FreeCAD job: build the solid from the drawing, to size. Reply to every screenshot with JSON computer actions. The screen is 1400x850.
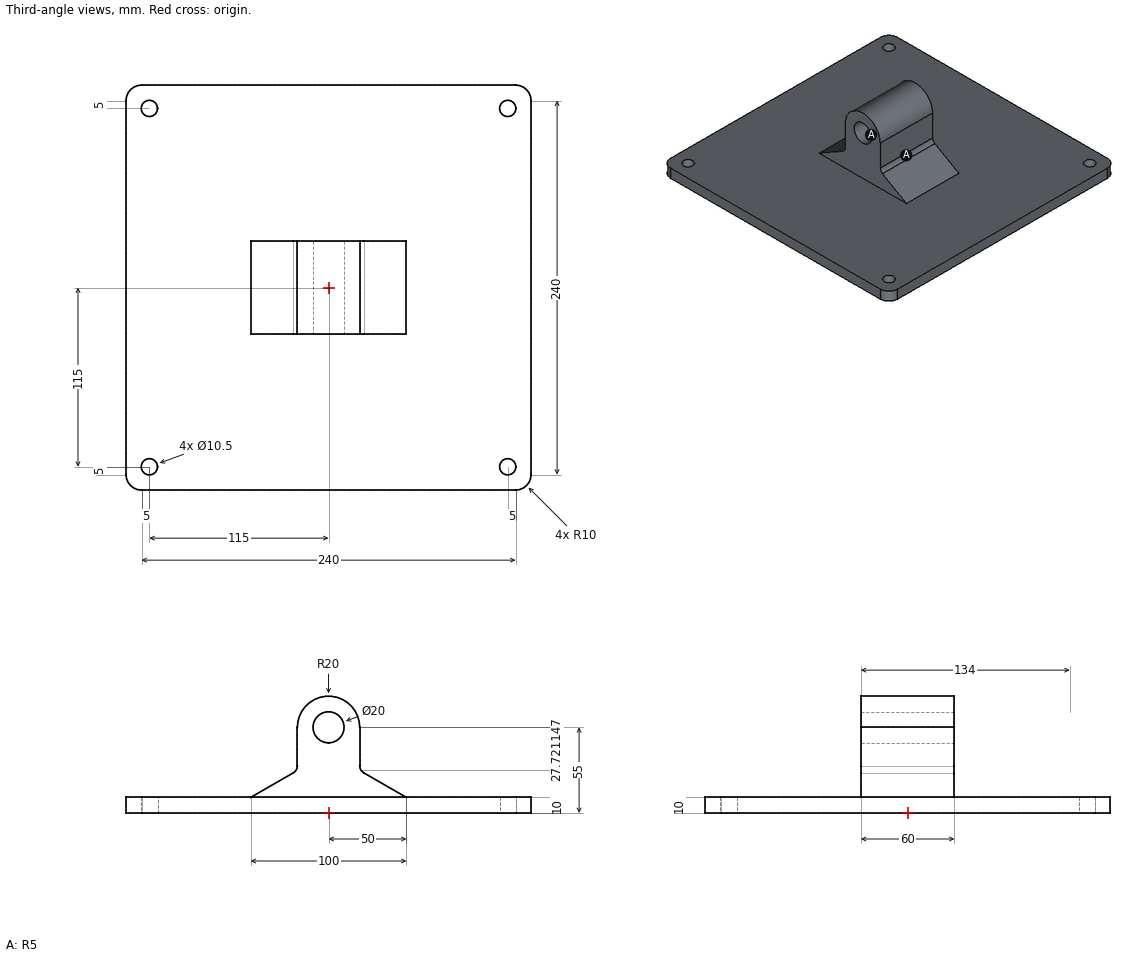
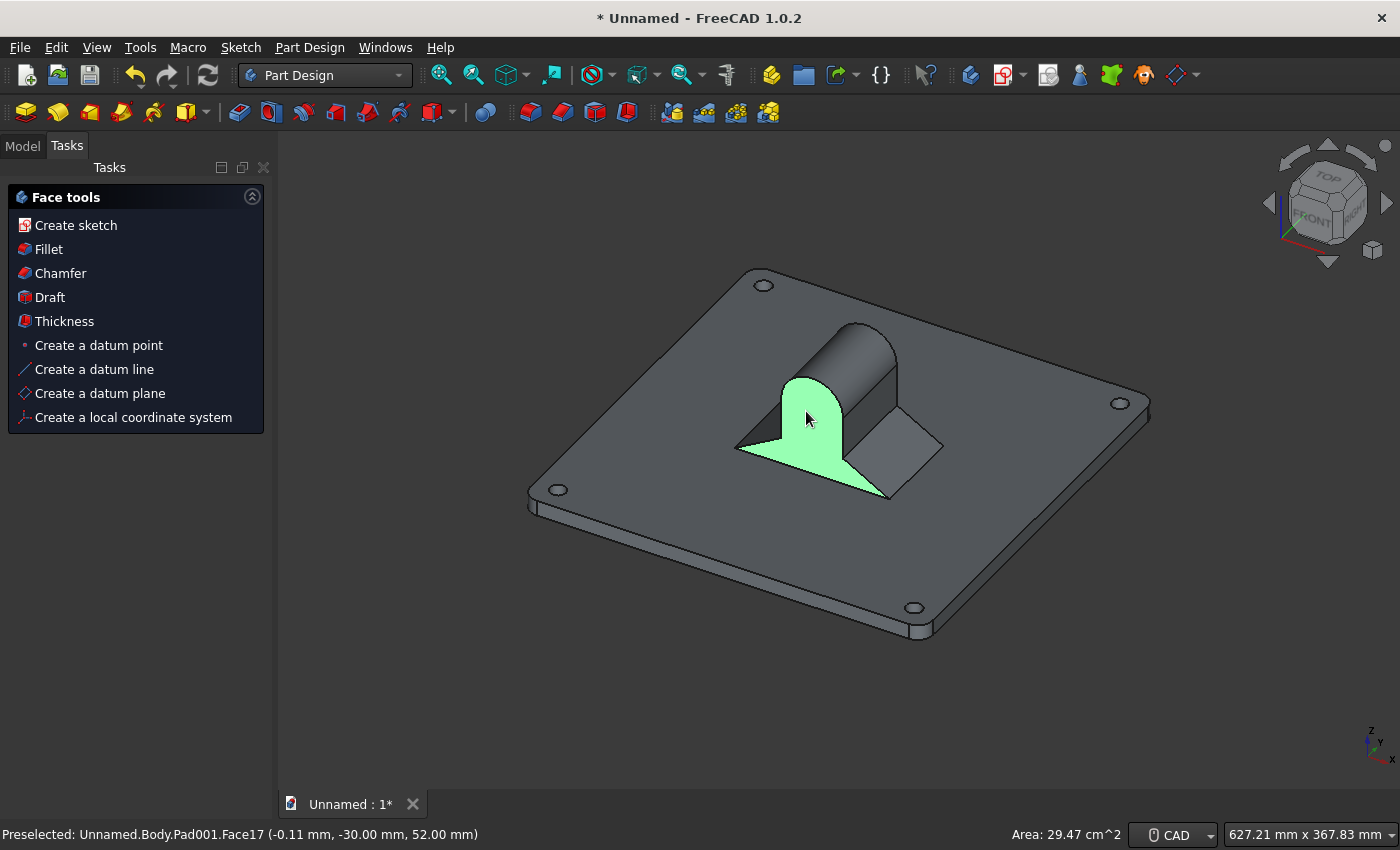
{"action": "left_click", "coordinate": [1004, 76]}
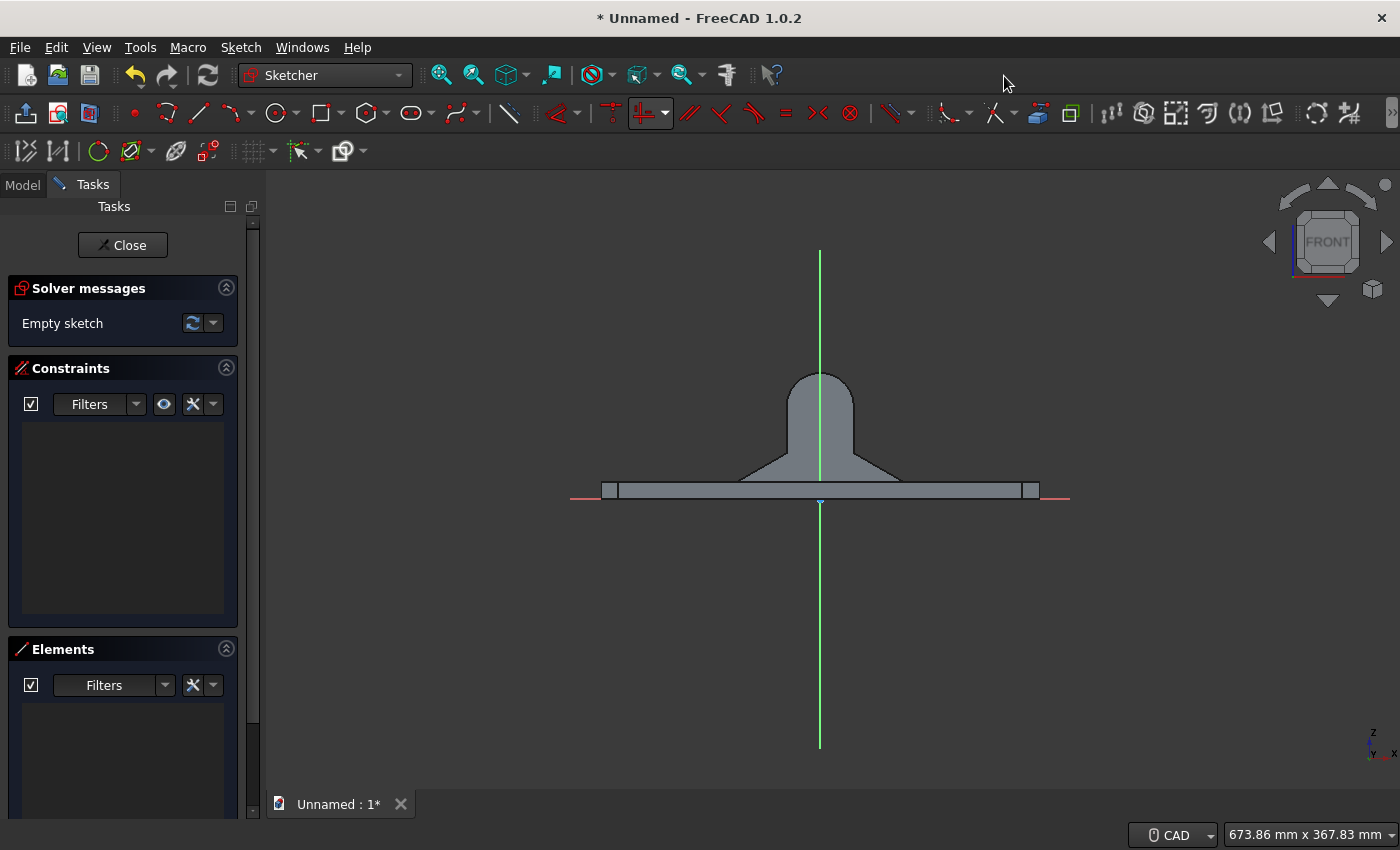
{"action": "left_click", "coordinate": [90, 114]}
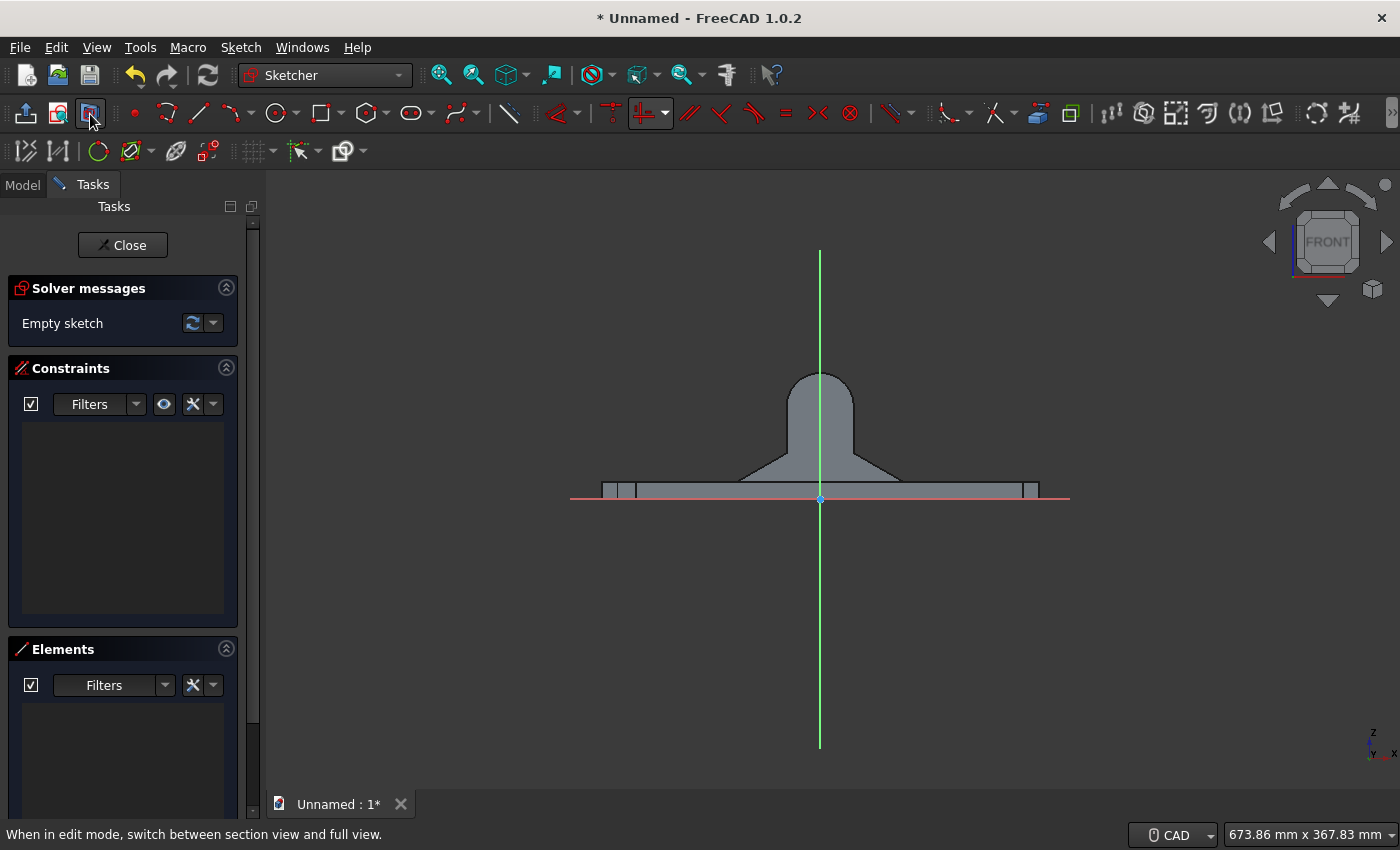
{"action": "scroll", "coordinate": [826, 399], "scroll_direction": "up", "scroll_amount": 12}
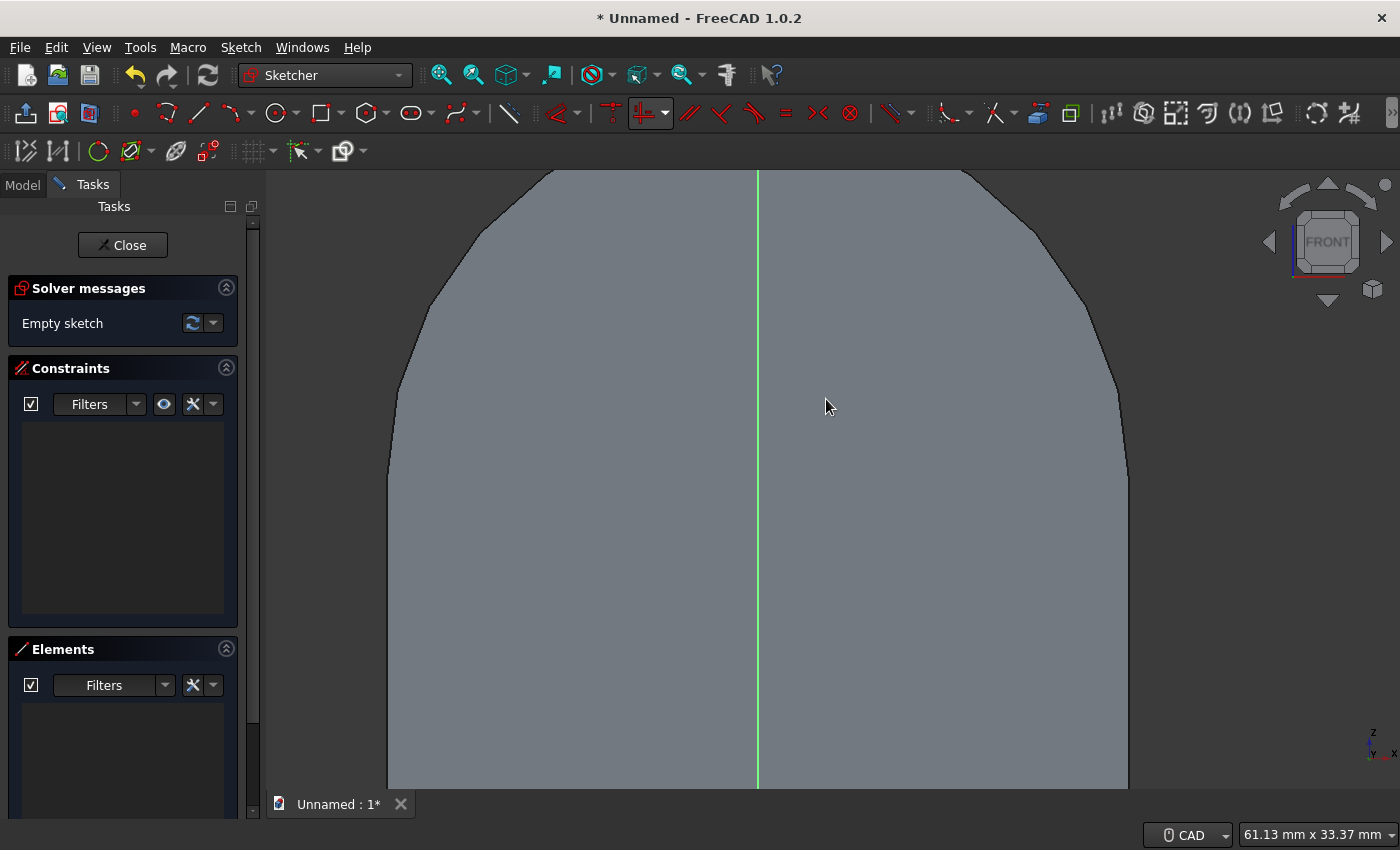
{"action": "left_click", "coordinate": [276, 114]}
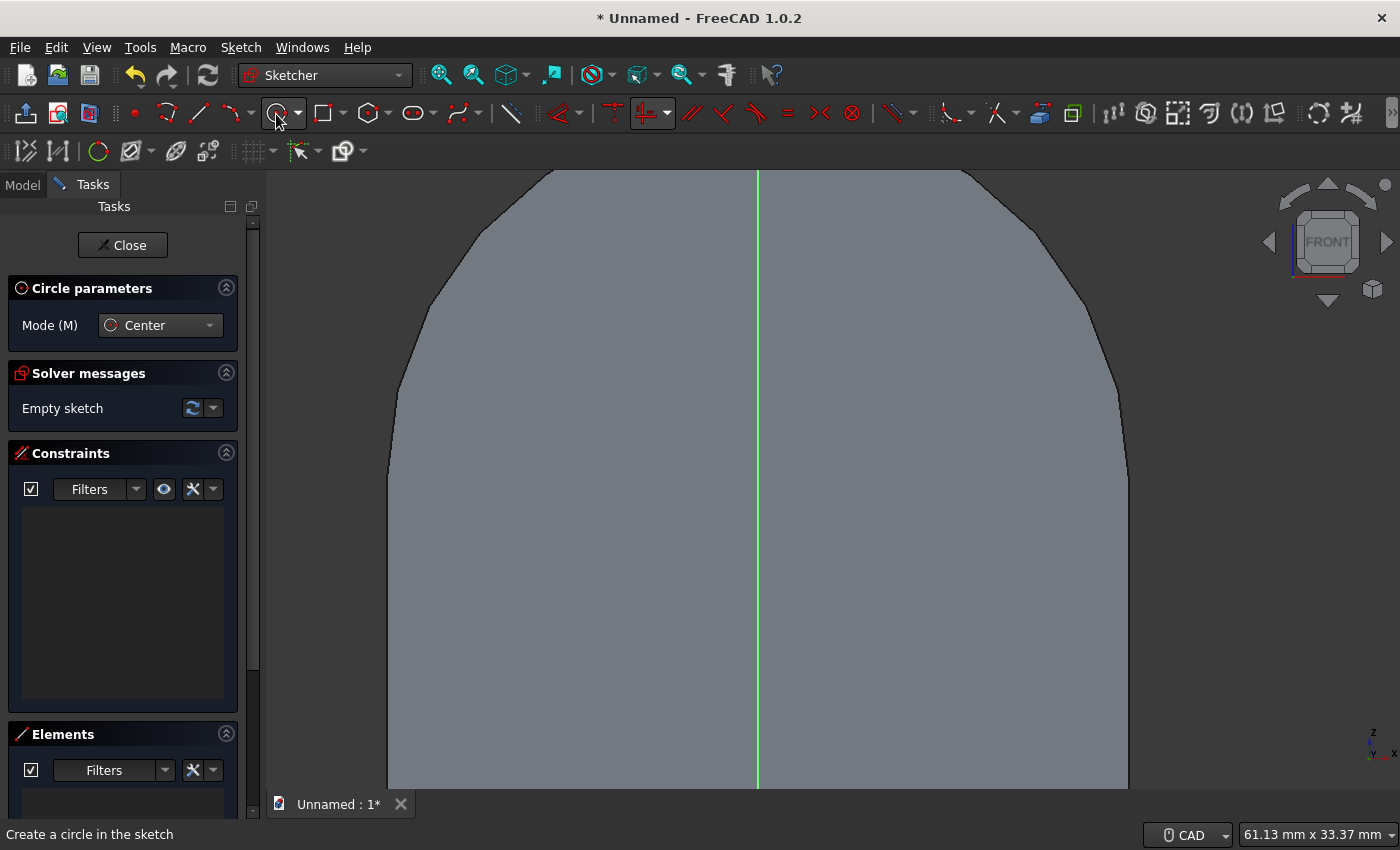
{"action": "left_click", "coordinate": [758, 479]}
{"action": "left_click", "coordinate": [889, 348]}
{"action": "key", "text": "Escape"}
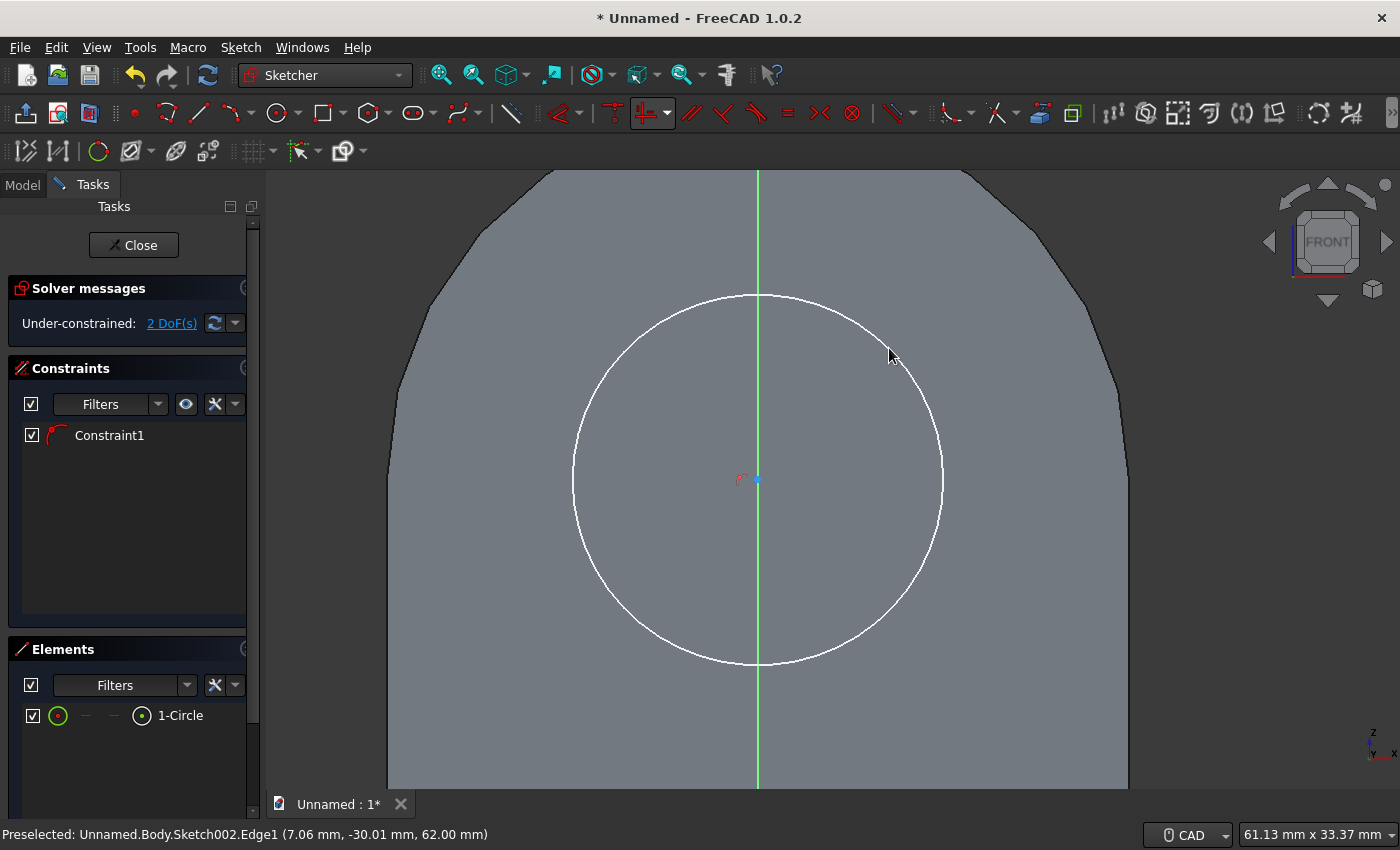
{"action": "left_click", "coordinate": [558, 114]}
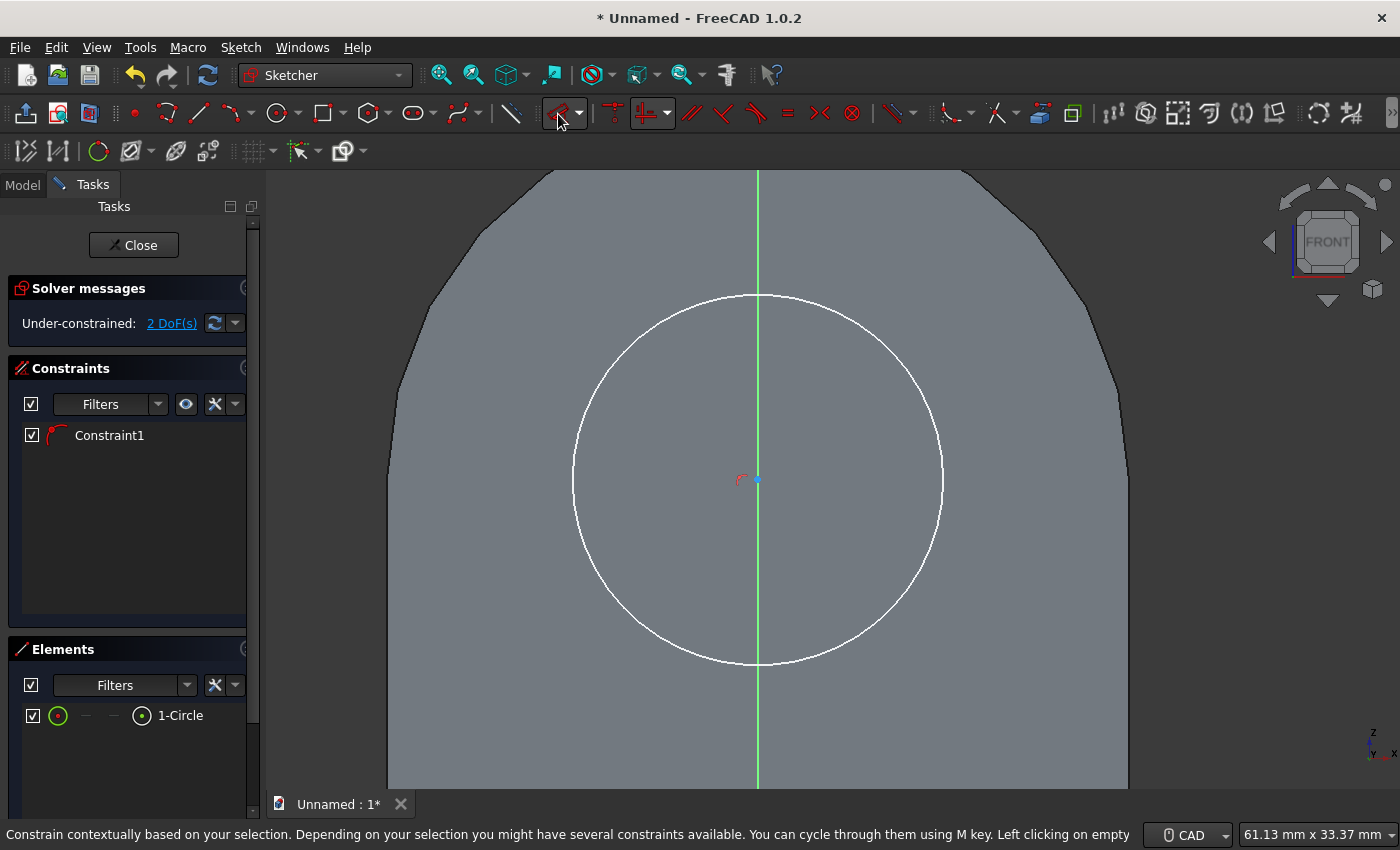
{"action": "left_click", "coordinate": [889, 349]}
{"action": "left_click", "coordinate": [912, 326]}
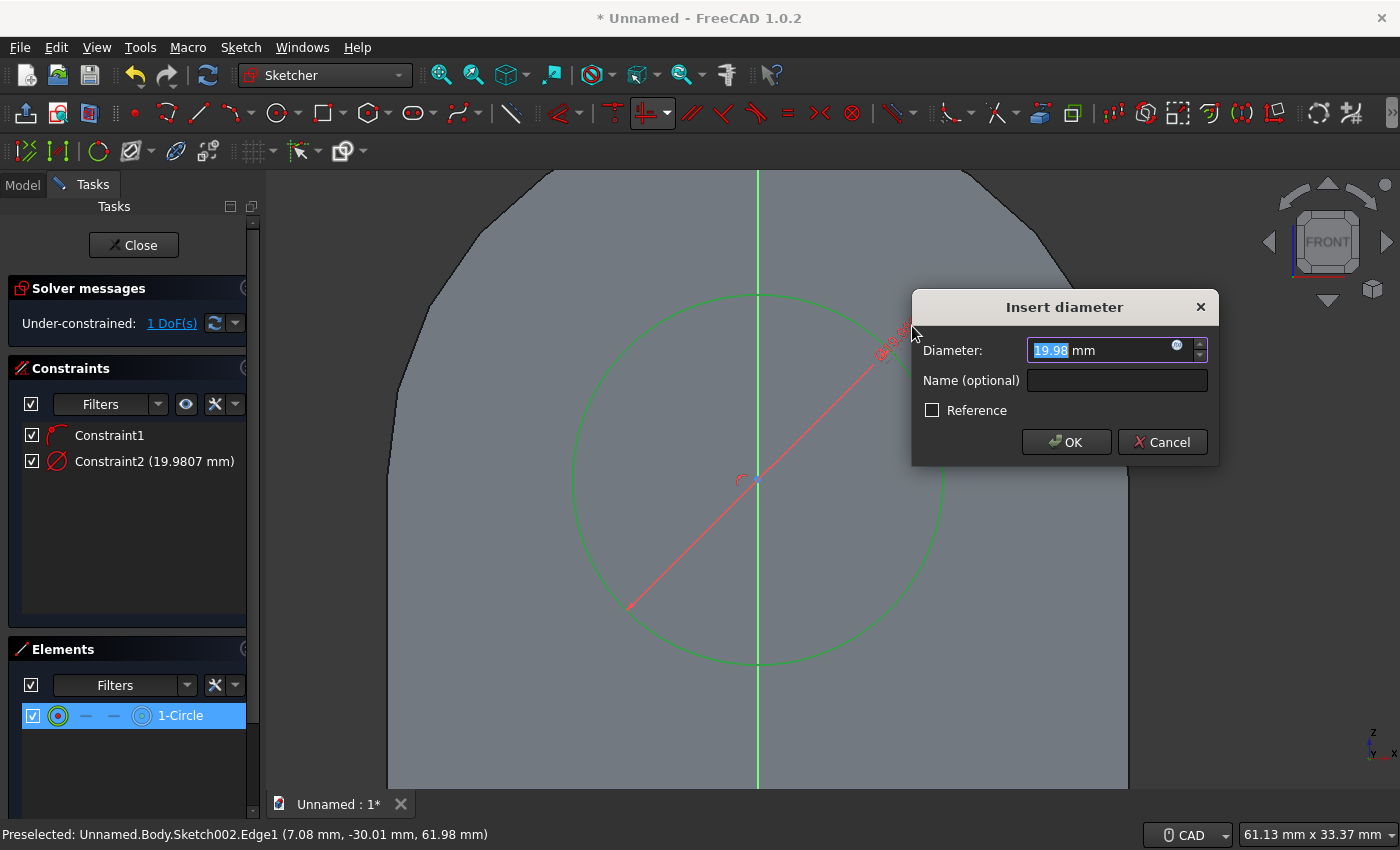
{"action": "type", "text": "20"}
{"action": "key", "text": "Return"}